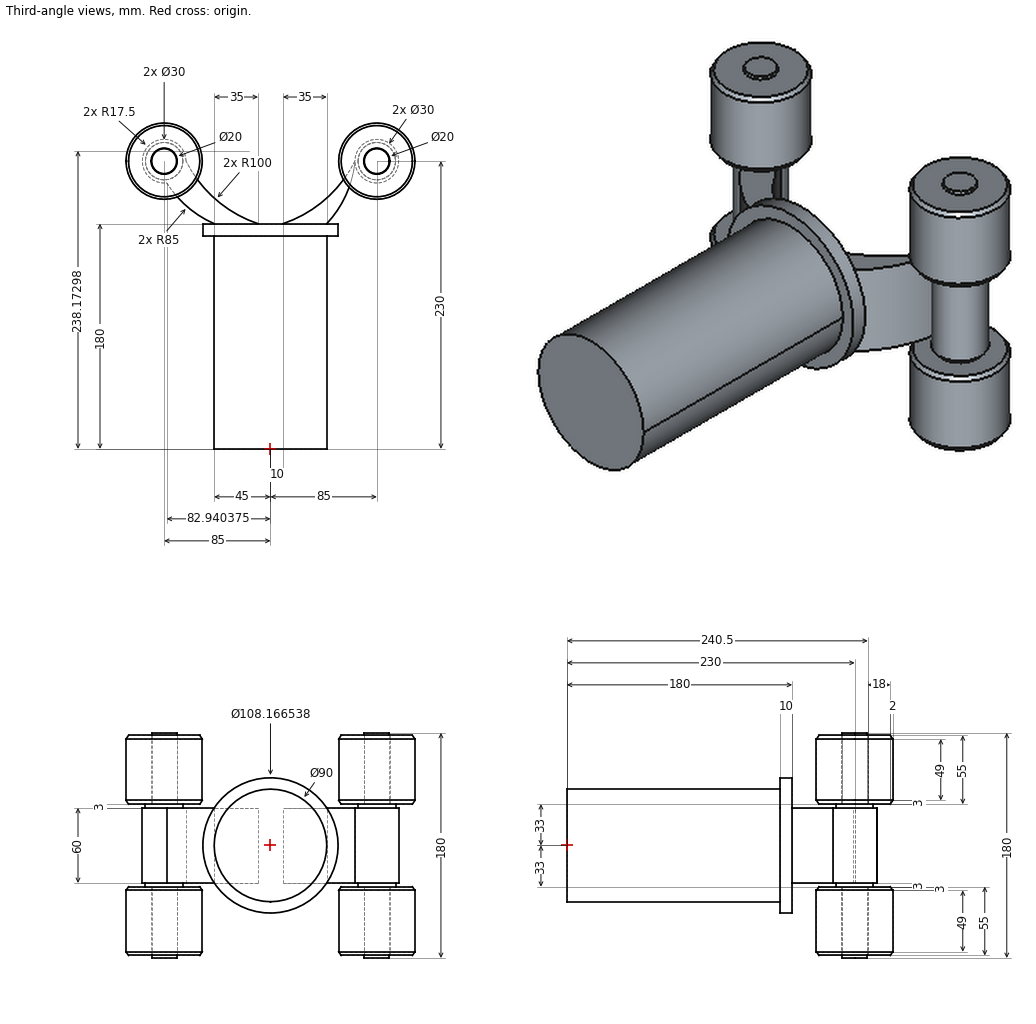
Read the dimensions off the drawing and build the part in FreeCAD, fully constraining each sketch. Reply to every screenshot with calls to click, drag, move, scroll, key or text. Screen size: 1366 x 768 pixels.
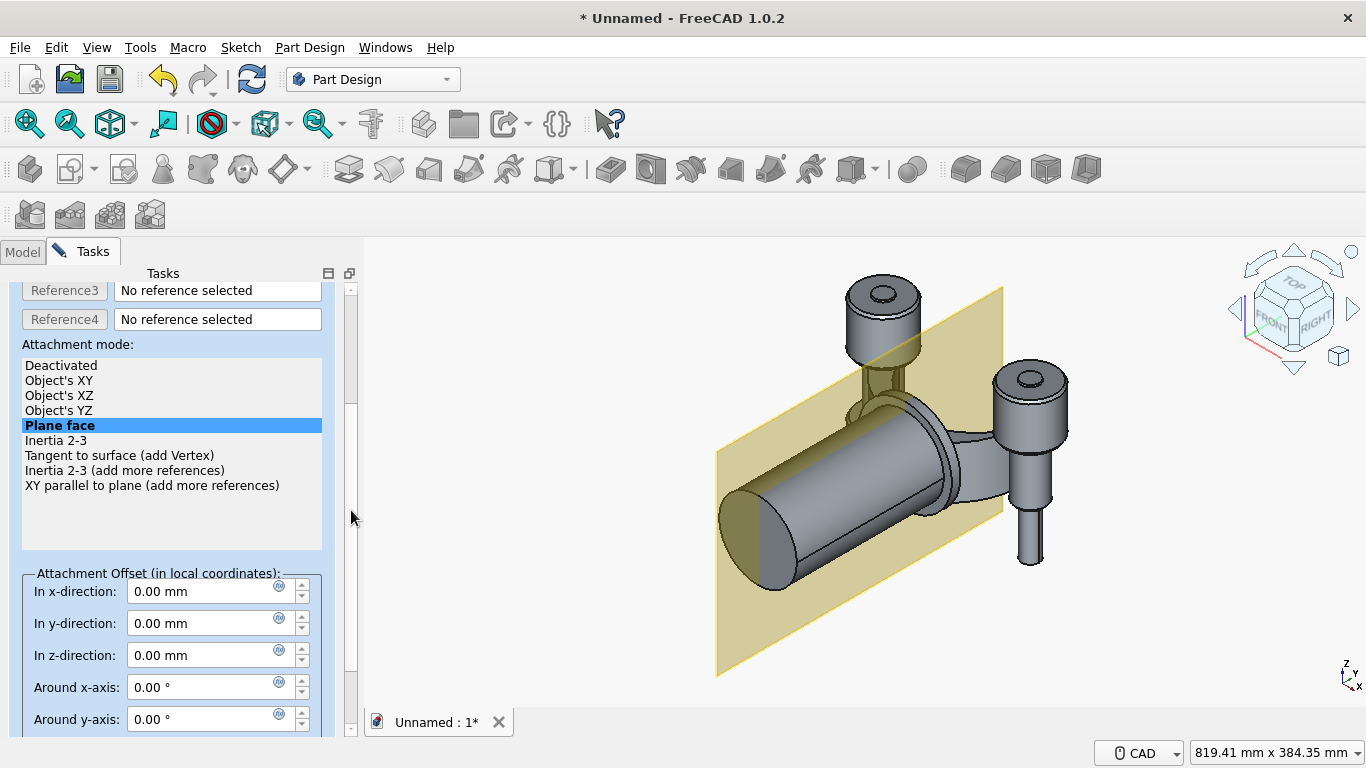
triple_click(210, 655)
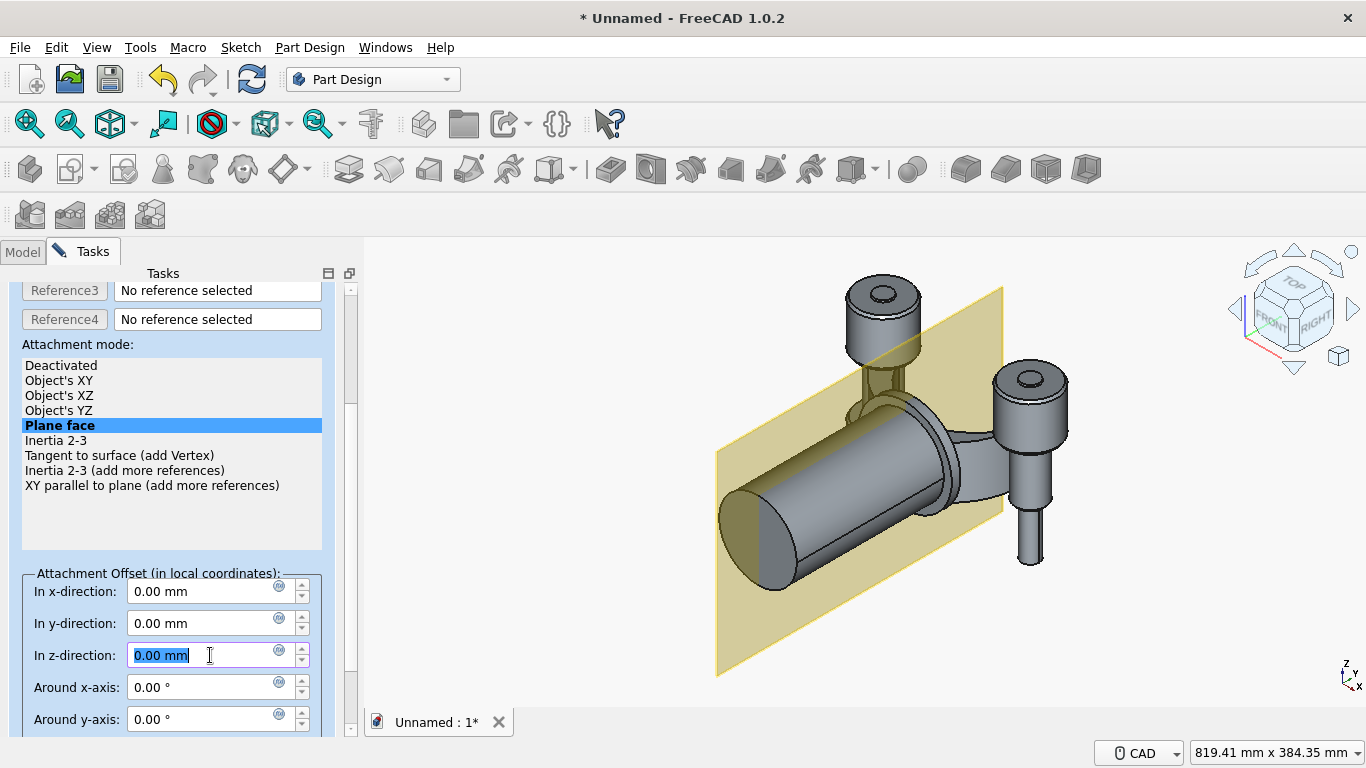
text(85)
key(Tab)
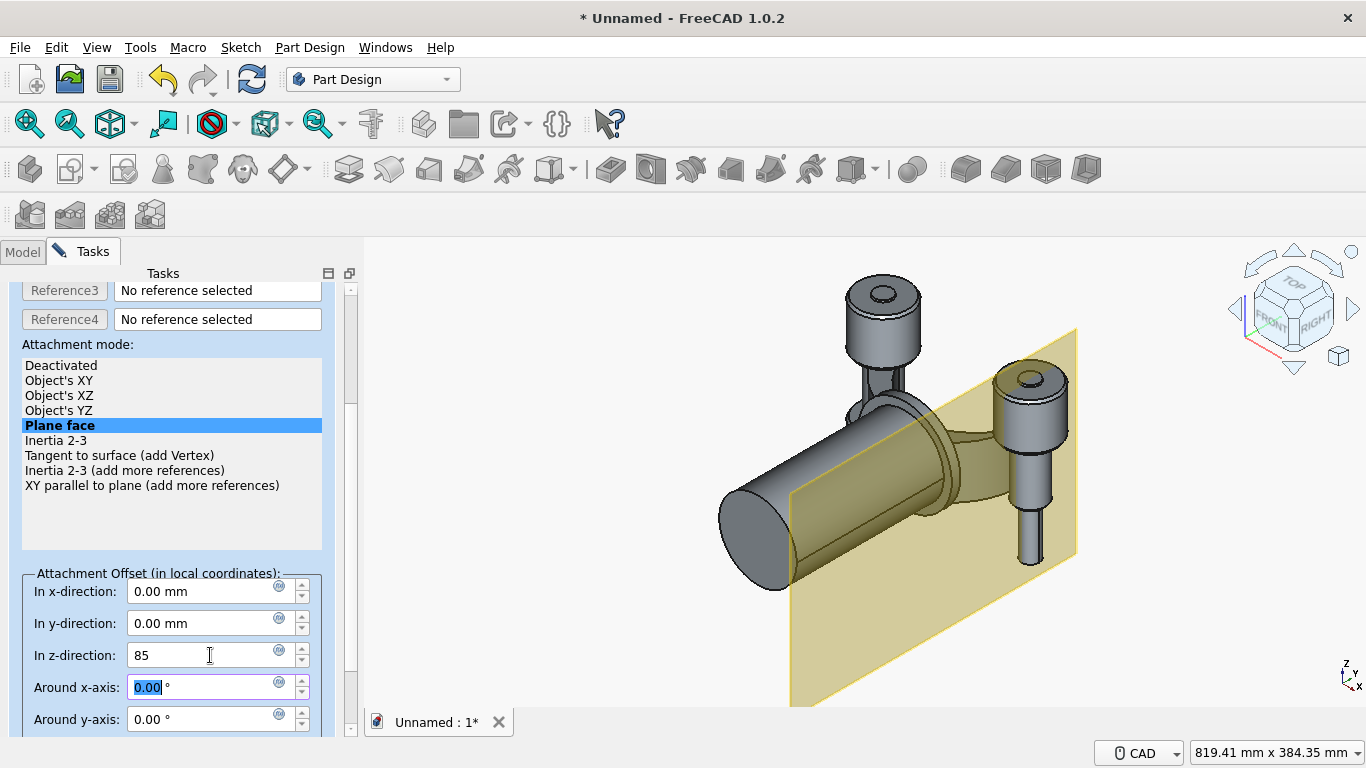
scroll(351, 510, up, 4)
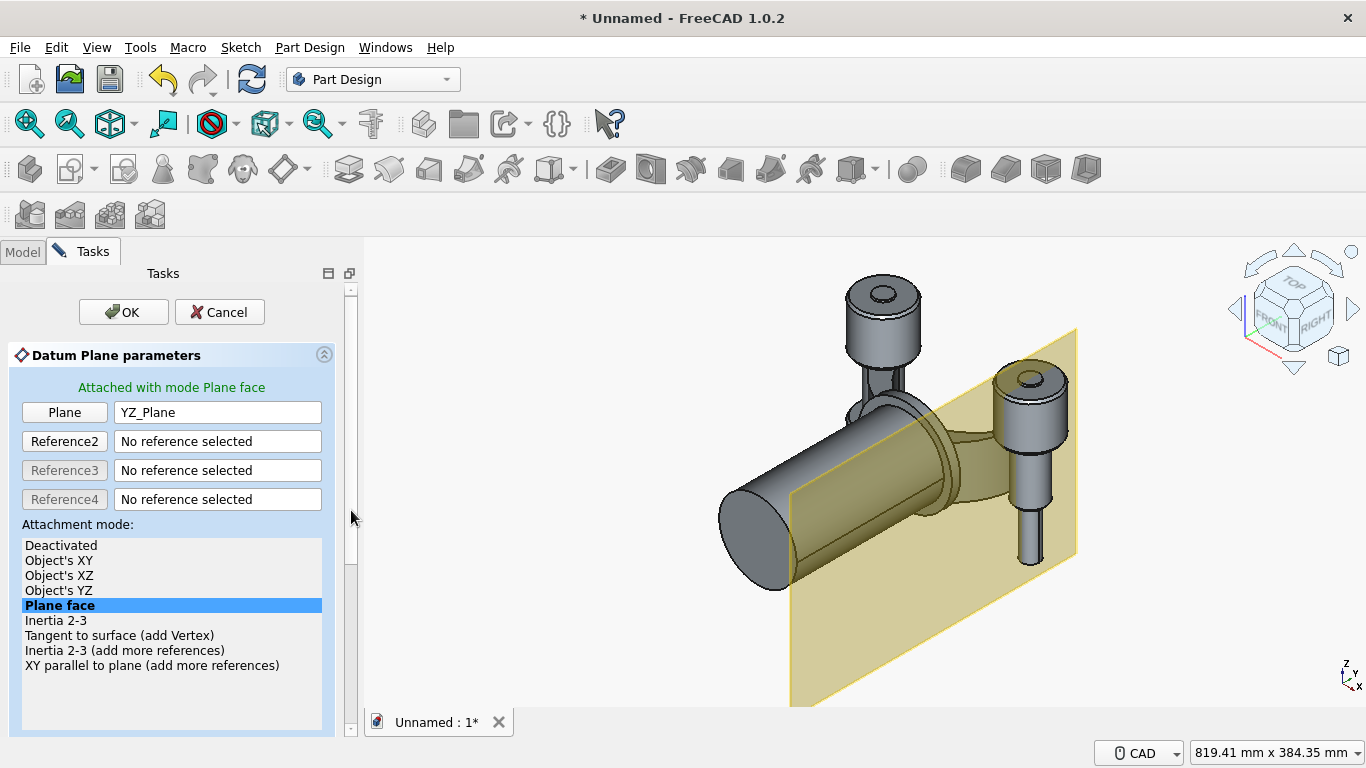
click(124, 312)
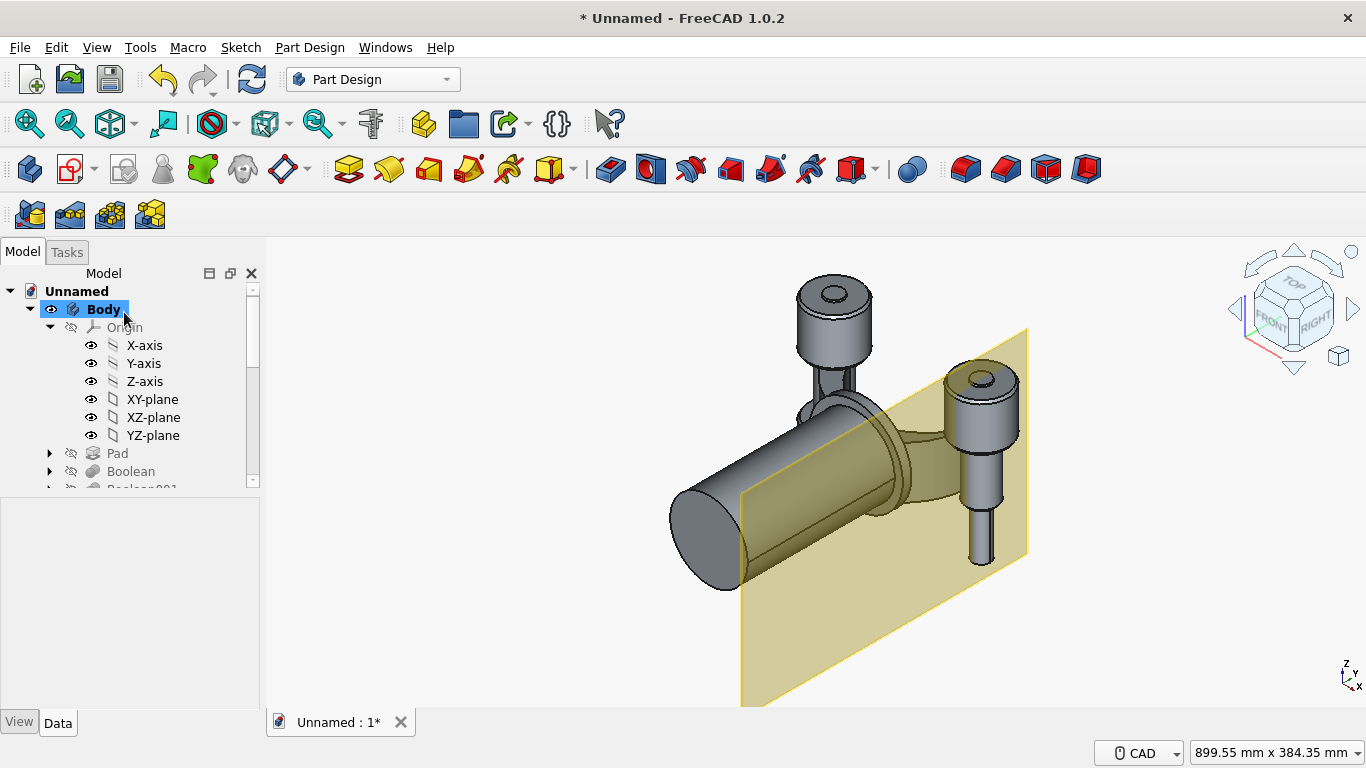
scroll(100, 377, down, 3)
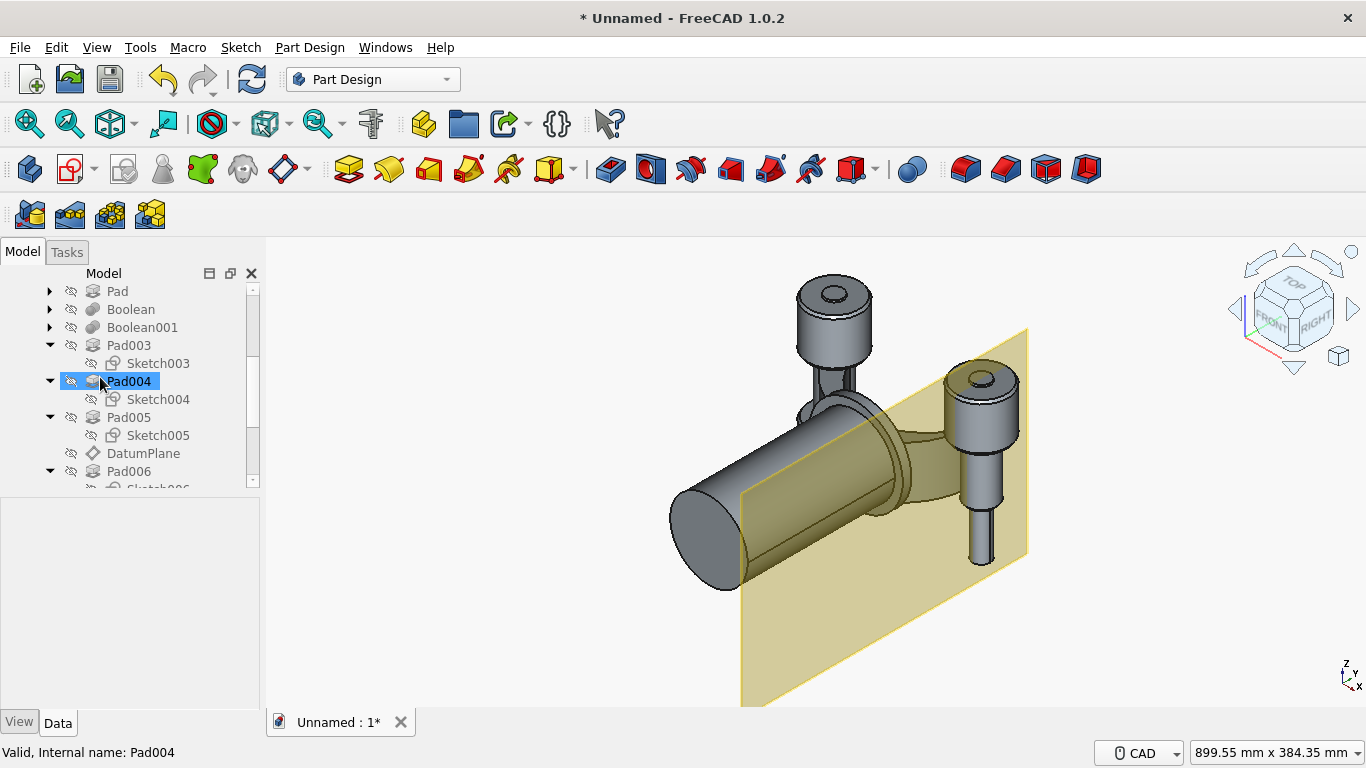
scroll(140, 377, up, 15)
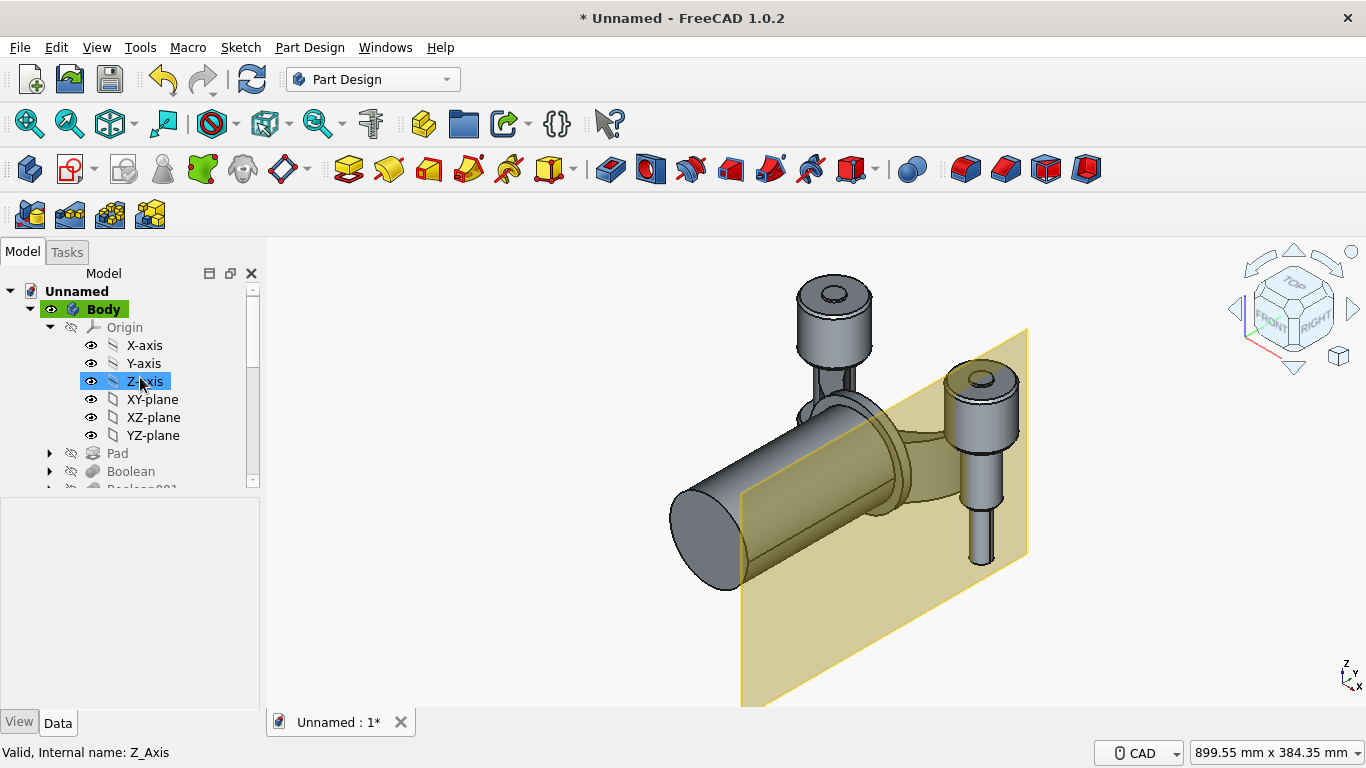
scroll(100, 377, down, 6)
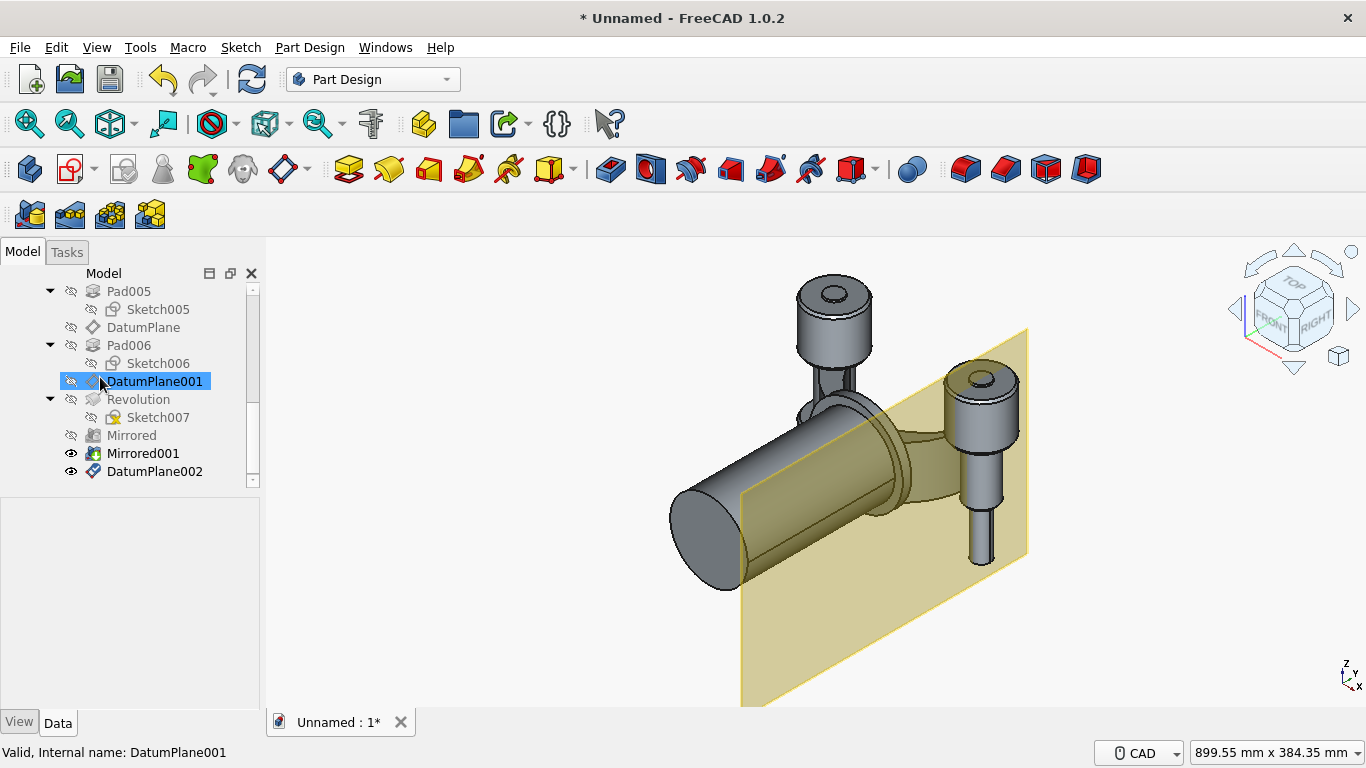
click(116, 471)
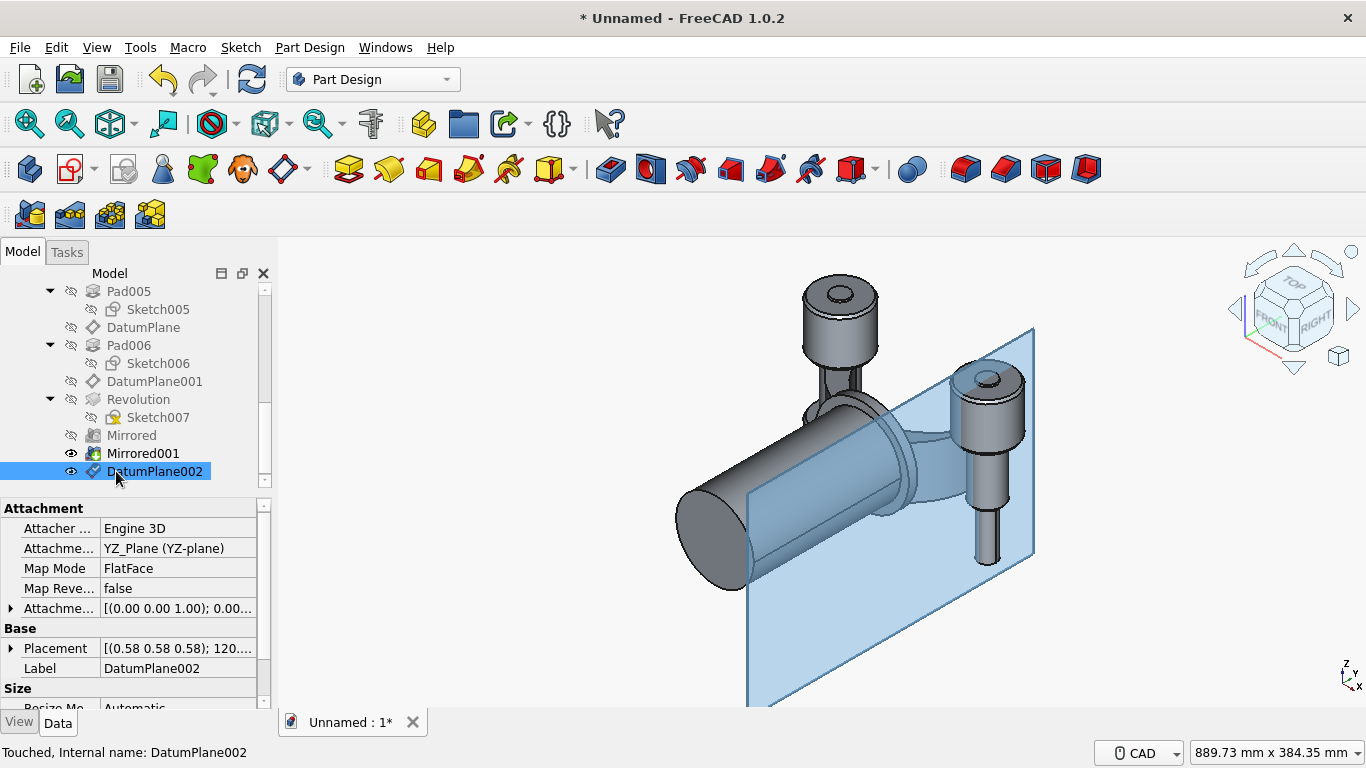
click(70, 170)